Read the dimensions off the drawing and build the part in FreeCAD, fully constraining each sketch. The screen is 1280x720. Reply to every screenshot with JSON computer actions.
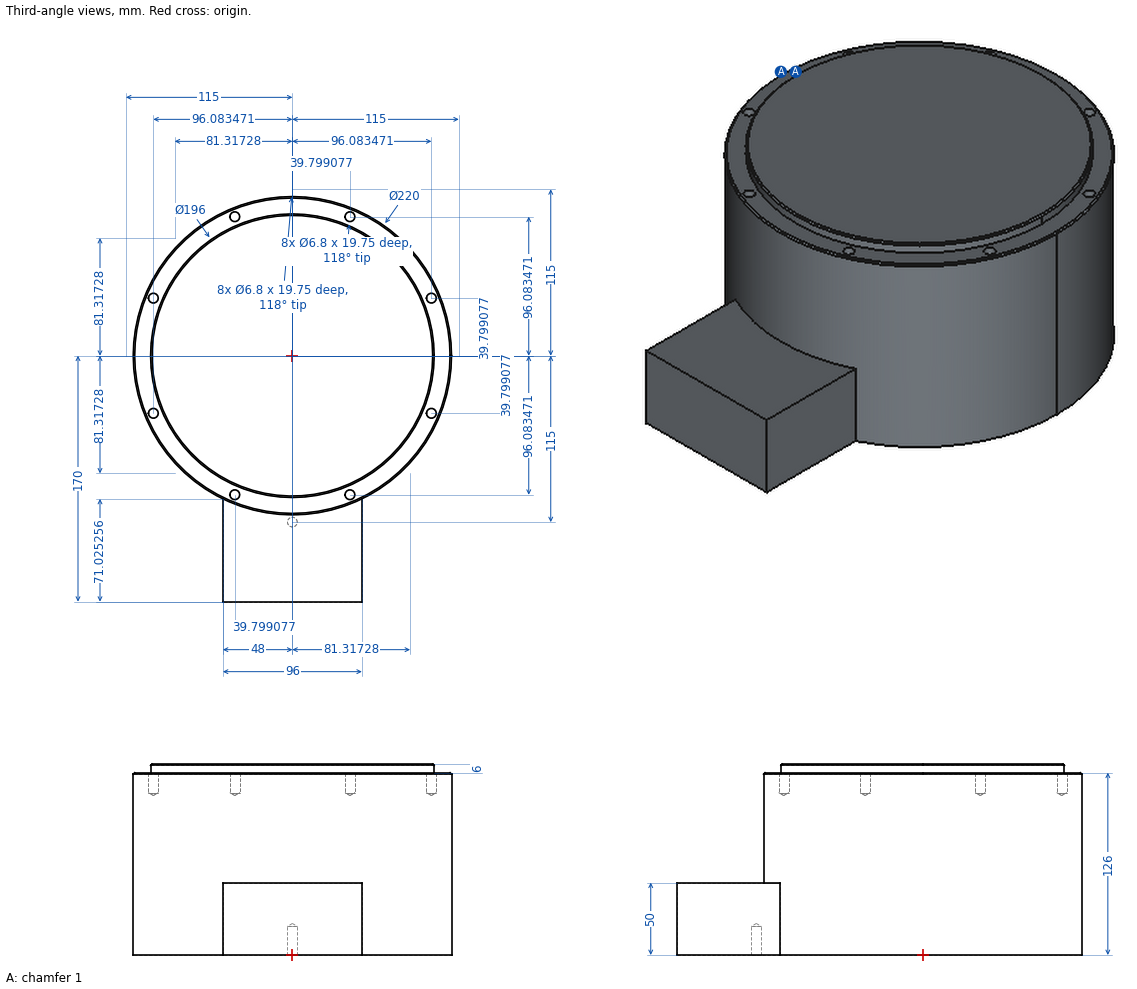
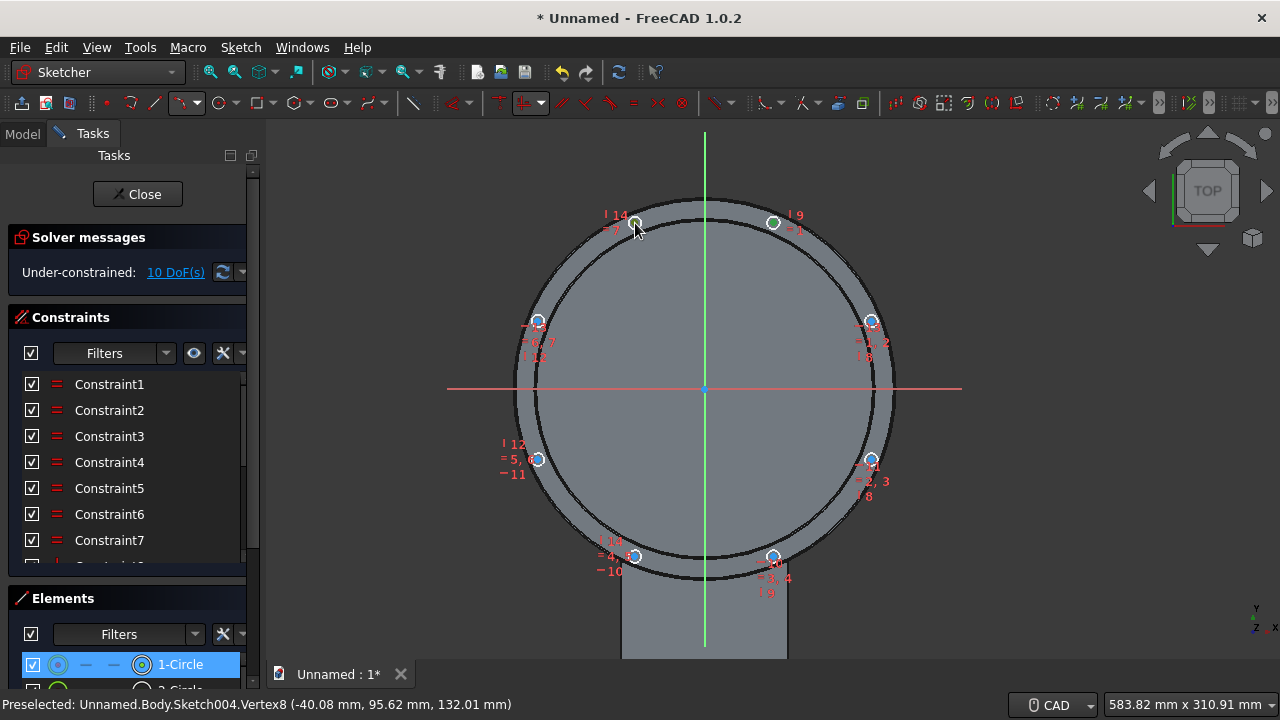
{"action": "left_click", "coordinate": [544, 104]}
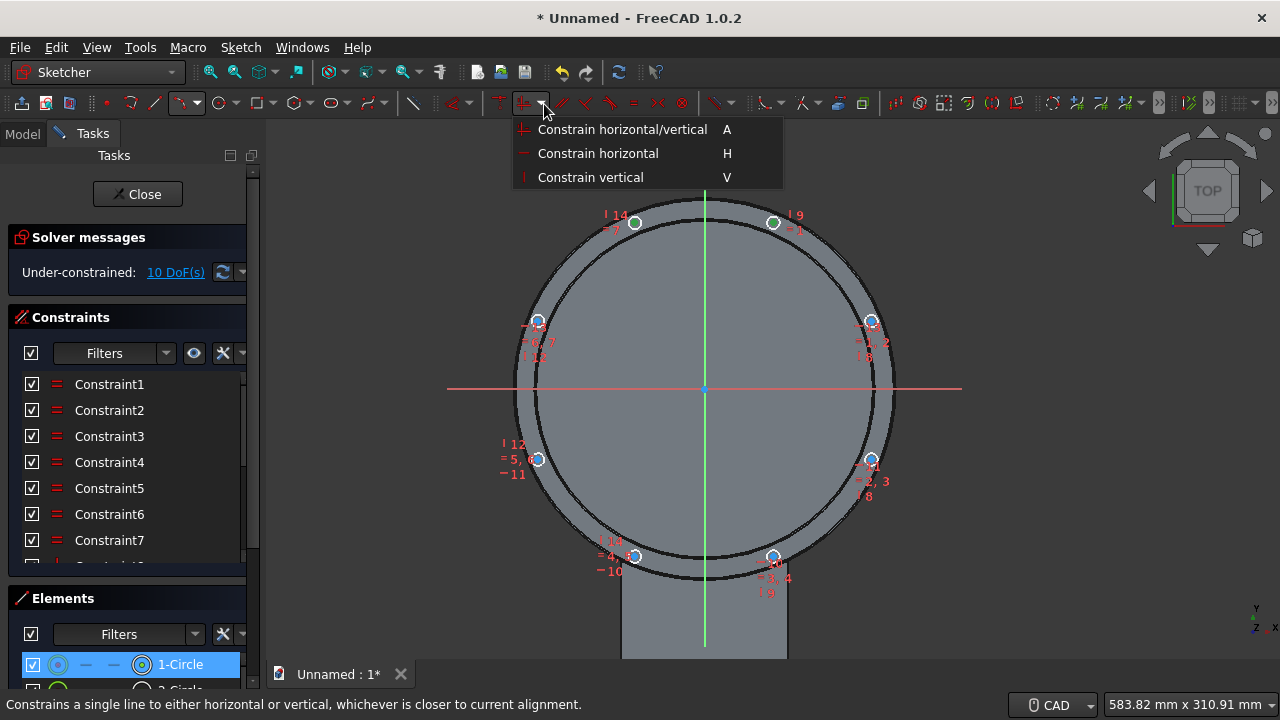
{"action": "left_click", "coordinate": [648, 153]}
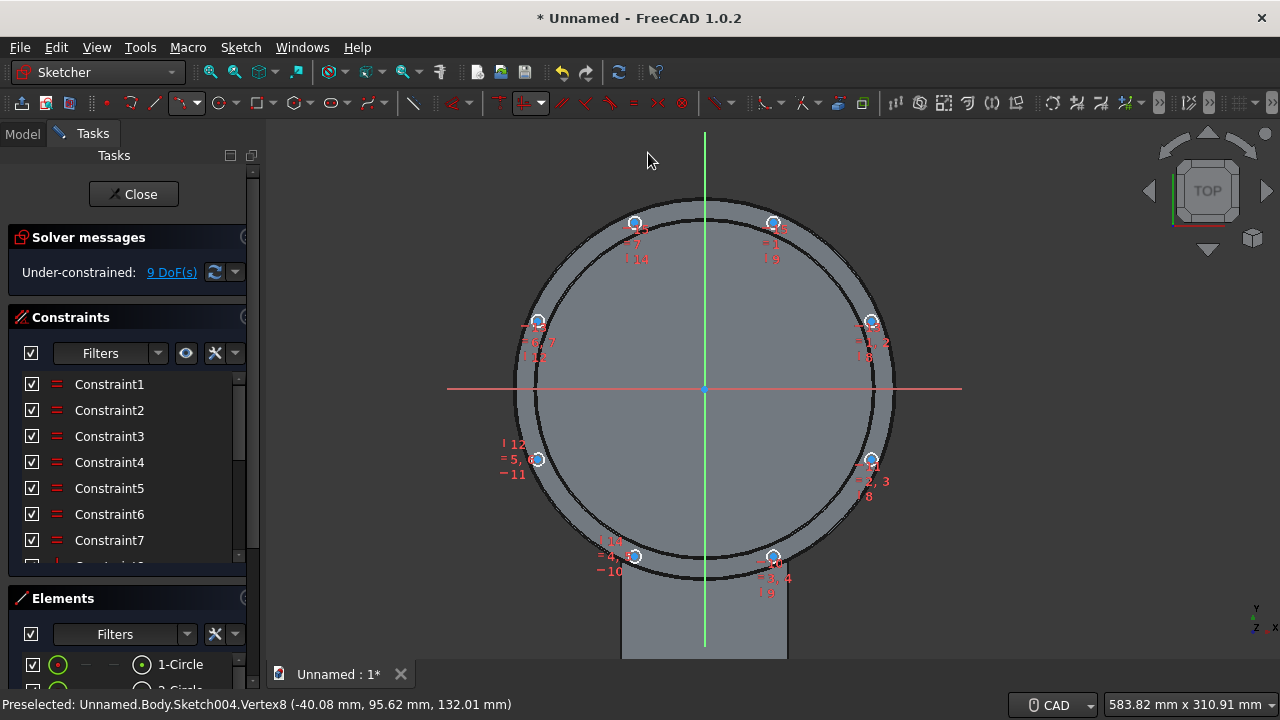
{"action": "left_click", "coordinate": [452, 104]}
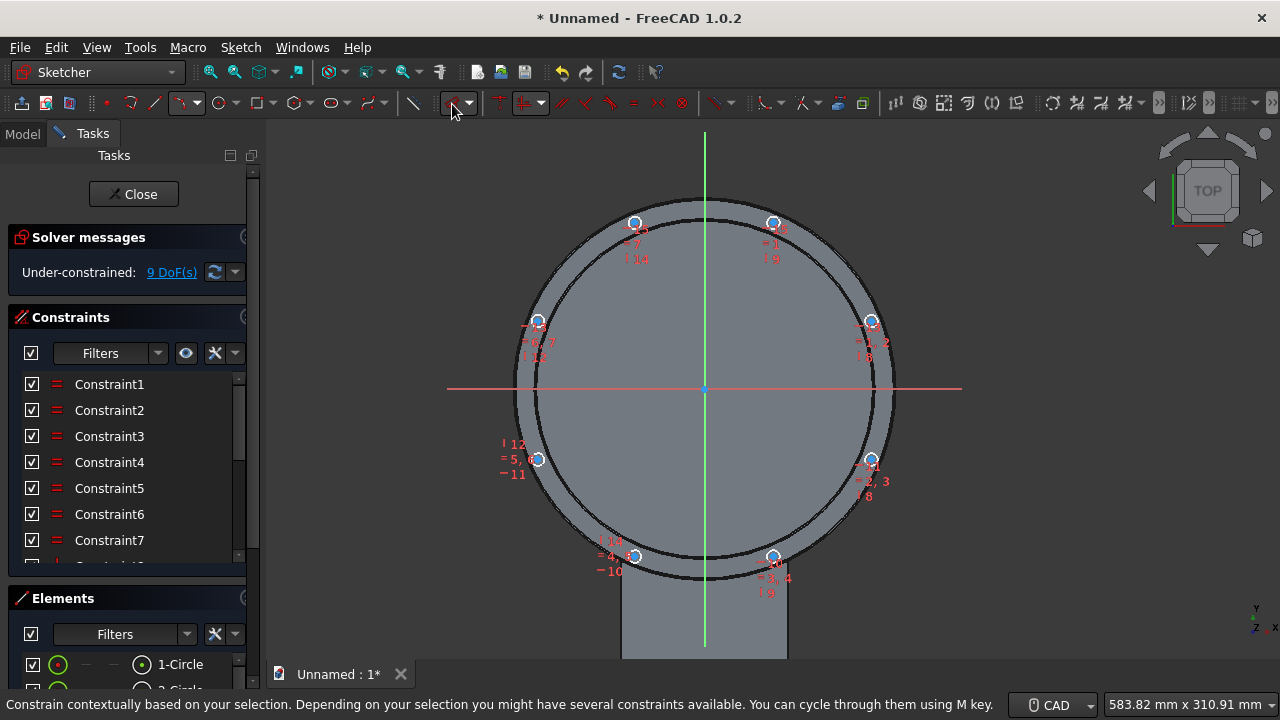
{"action": "scroll", "coordinate": [778, 227], "scroll_direction": "up", "scroll_amount": 7}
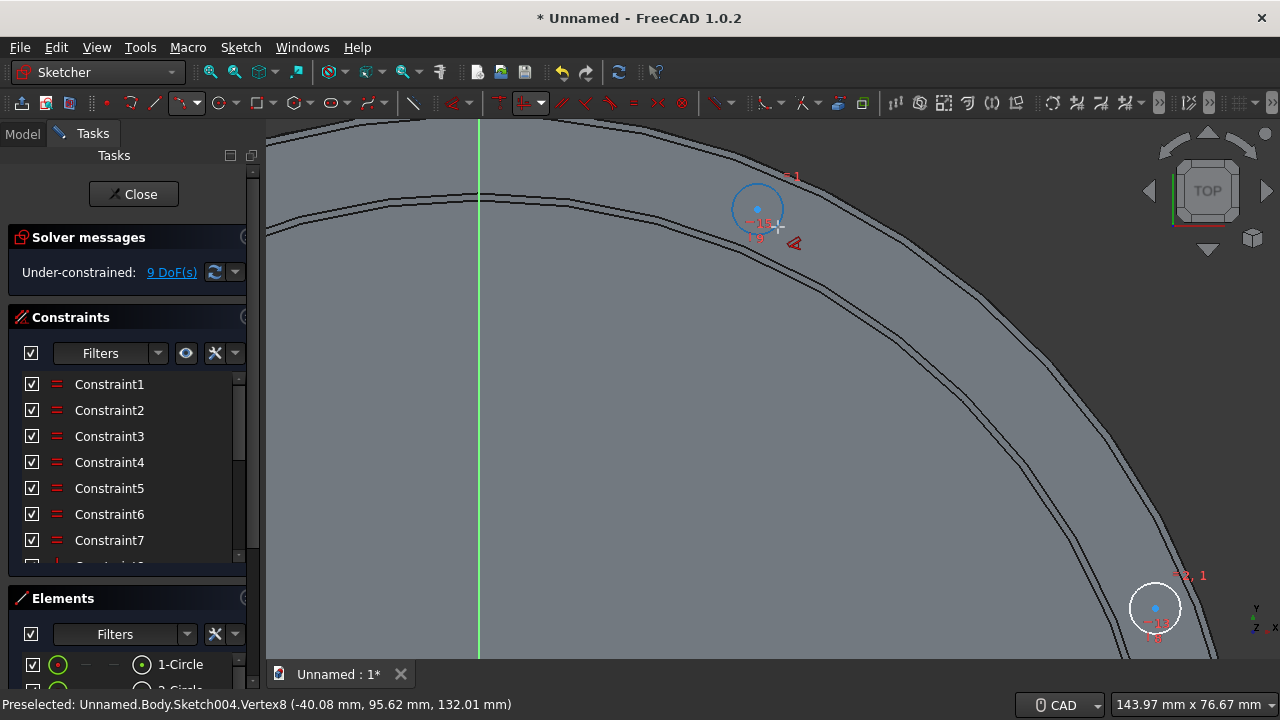
{"action": "left_click", "coordinate": [776, 227]}
{"action": "left_click", "coordinate": [799, 249]}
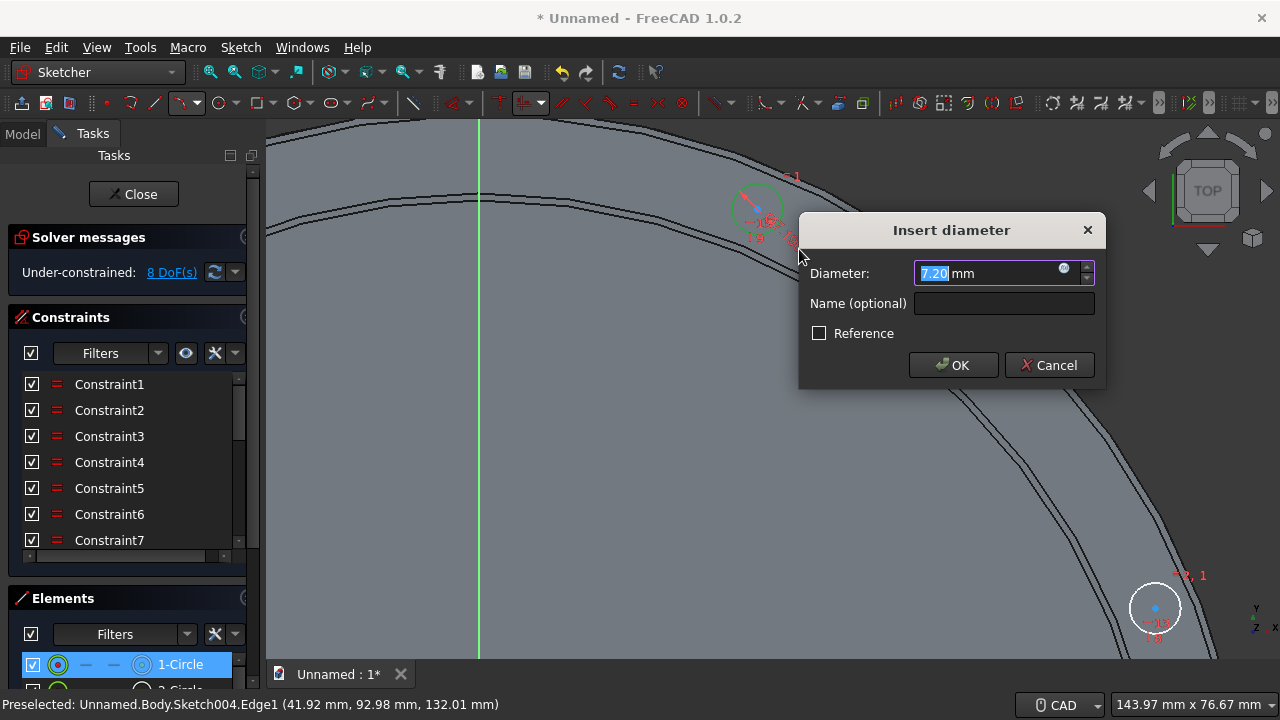
{"action": "type", "text": "6.8"}
{"action": "key", "text": "Return"}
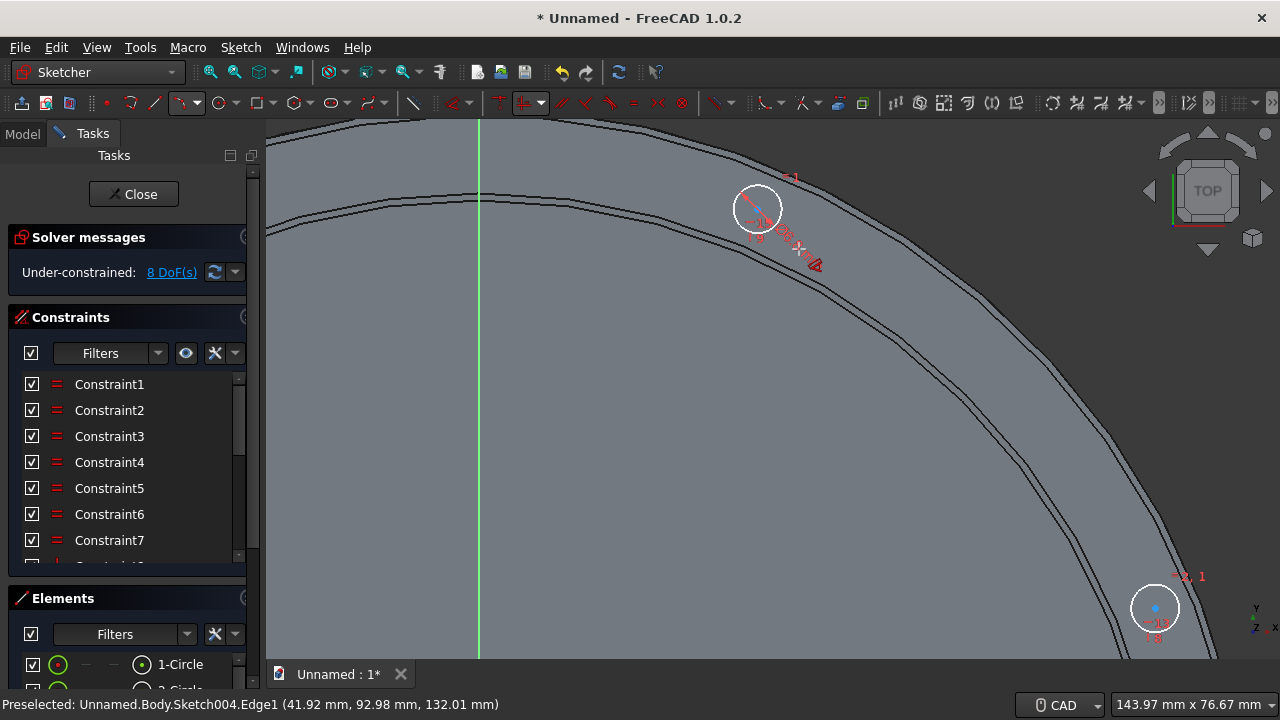
{"action": "scroll", "coordinate": [778, 227], "scroll_direction": "down", "scroll_amount": 7}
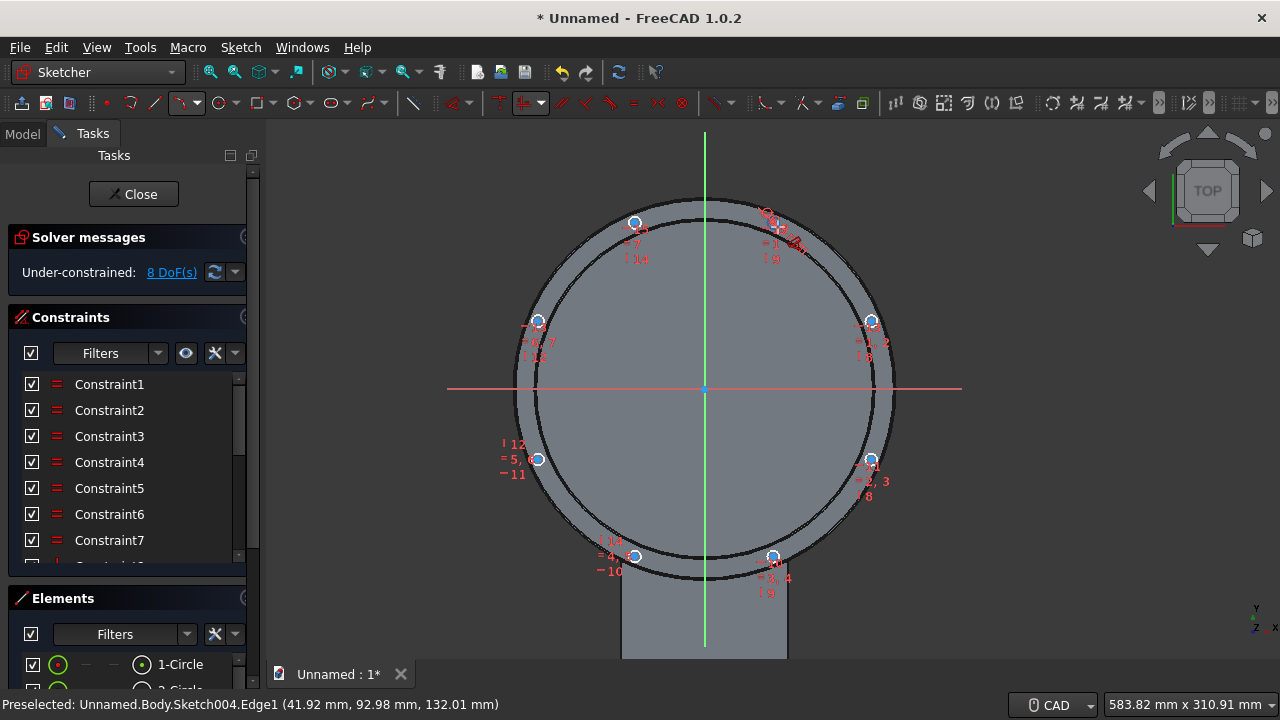
{"action": "left_click", "coordinate": [773, 223]}
{"action": "left_click", "coordinate": [739, 189]}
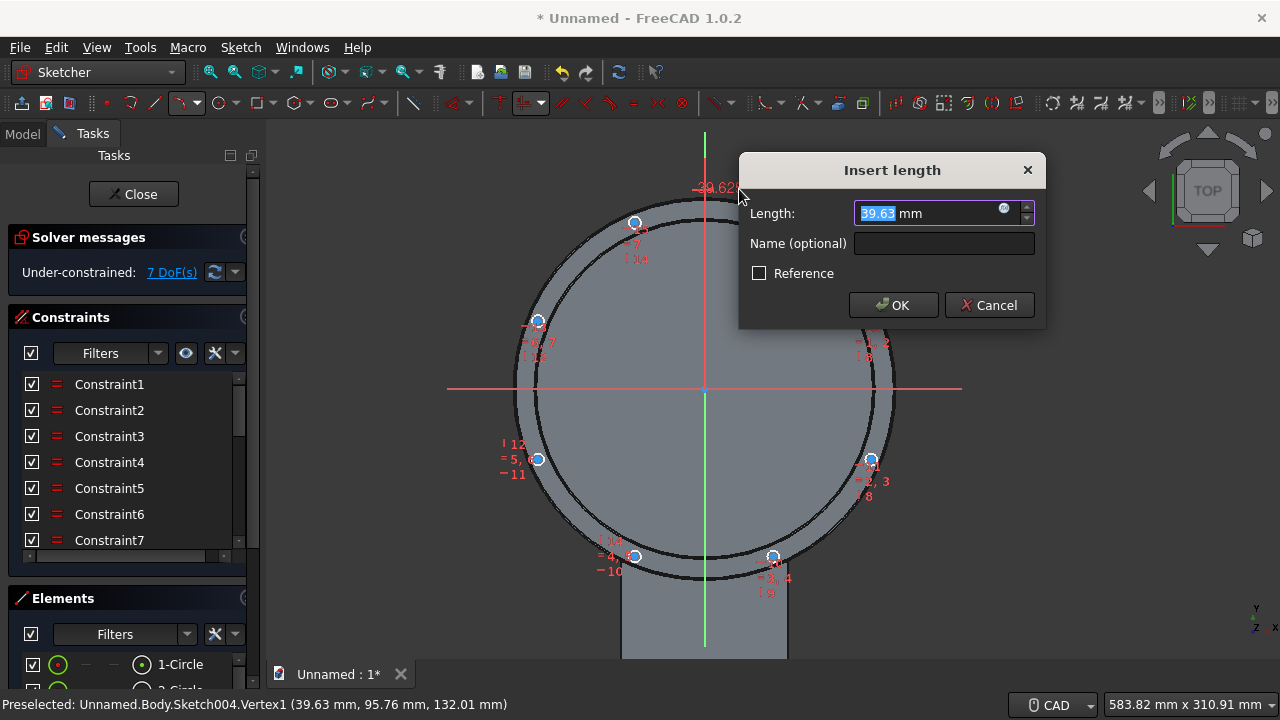
{"action": "type", "text": "39.799077"}
{"action": "key", "text": "Return"}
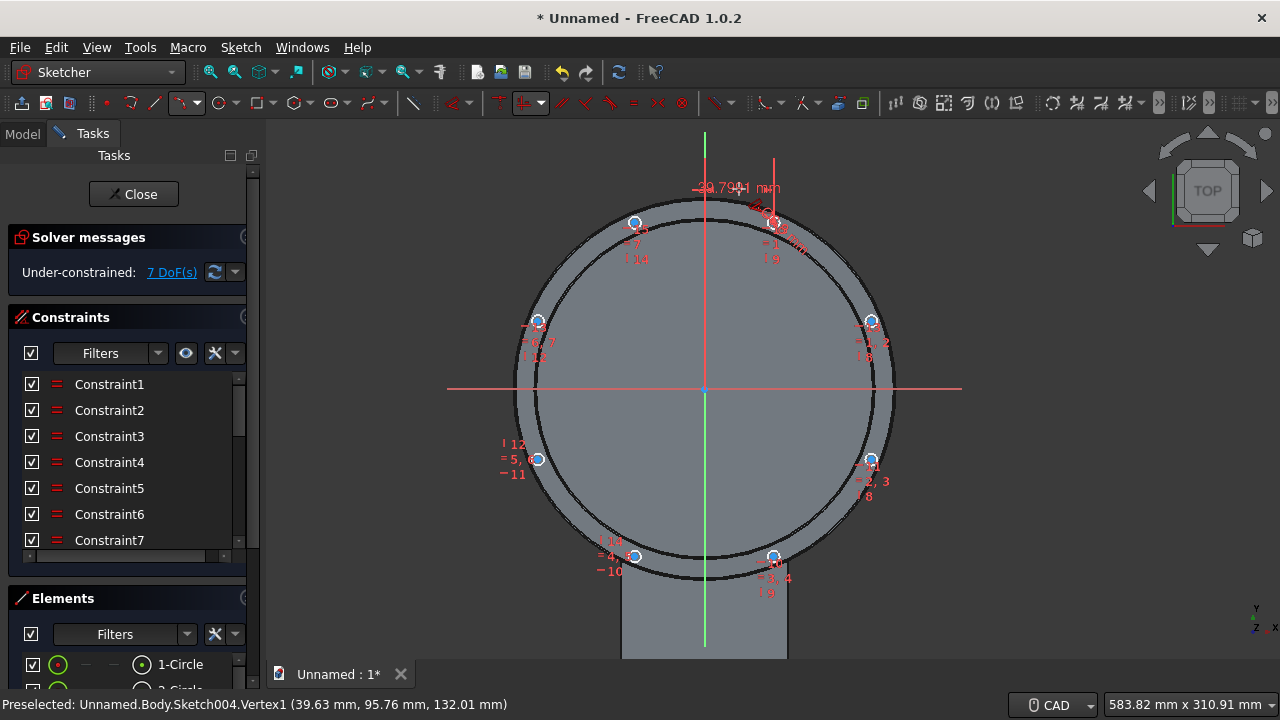
{"action": "left_click", "coordinate": [774, 223]}
{"action": "left_click", "coordinate": [808, 306]}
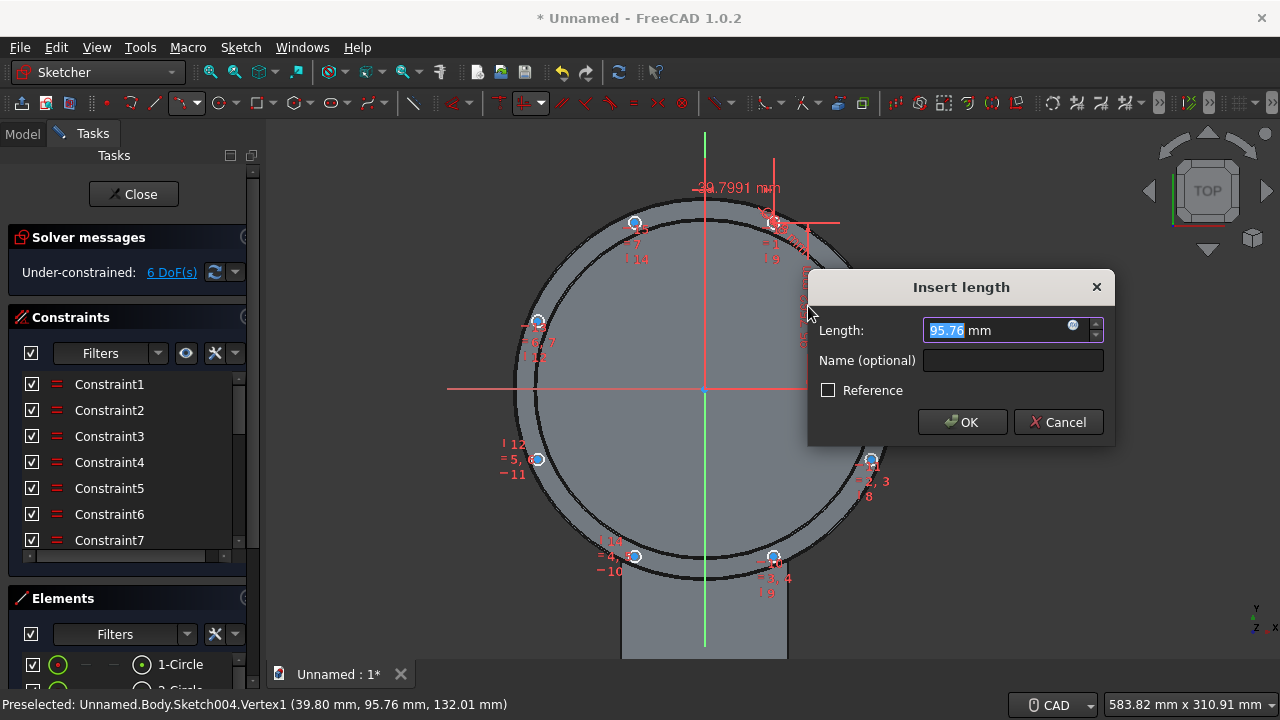
{"action": "type", "text": "96.083471"}
{"action": "key", "text": "Return"}